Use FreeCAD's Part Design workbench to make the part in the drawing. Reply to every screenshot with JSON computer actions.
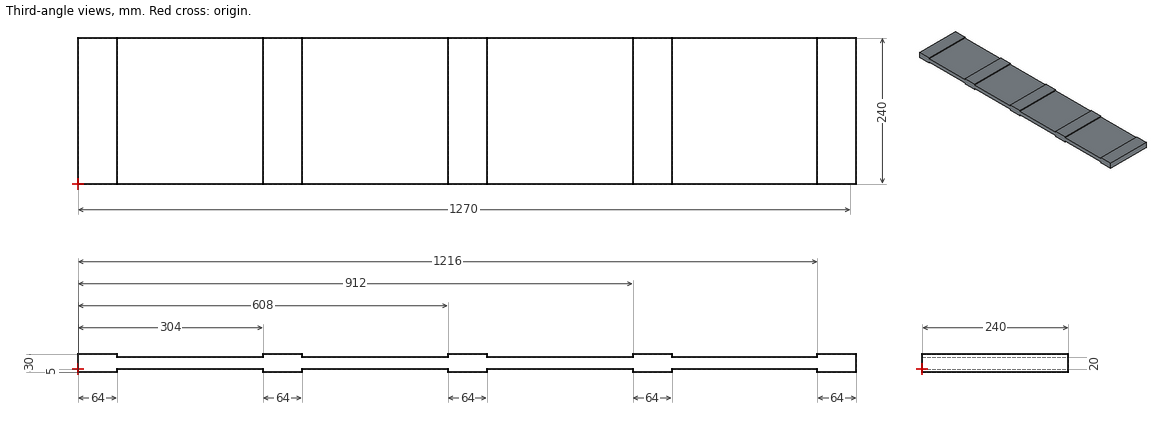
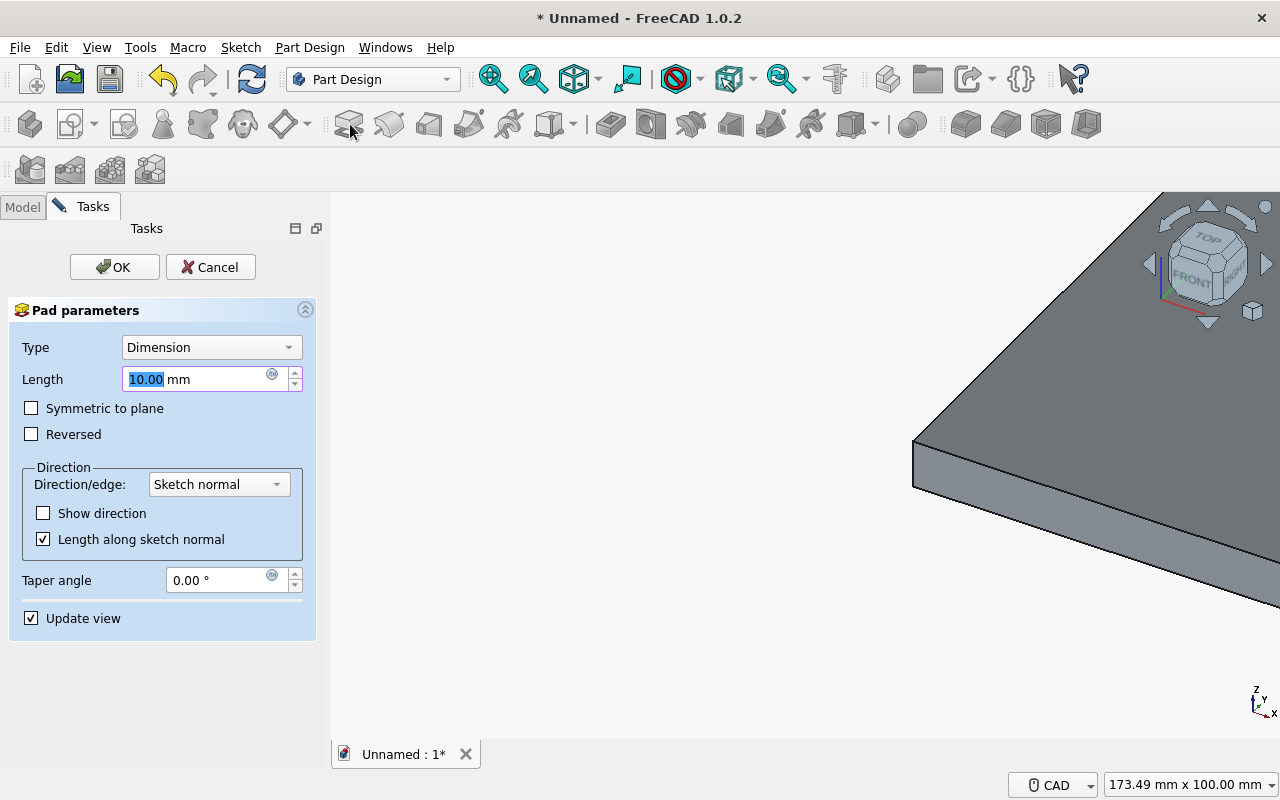
{"action": "type", "text": "20"}
{"action": "key", "text": "Tab"}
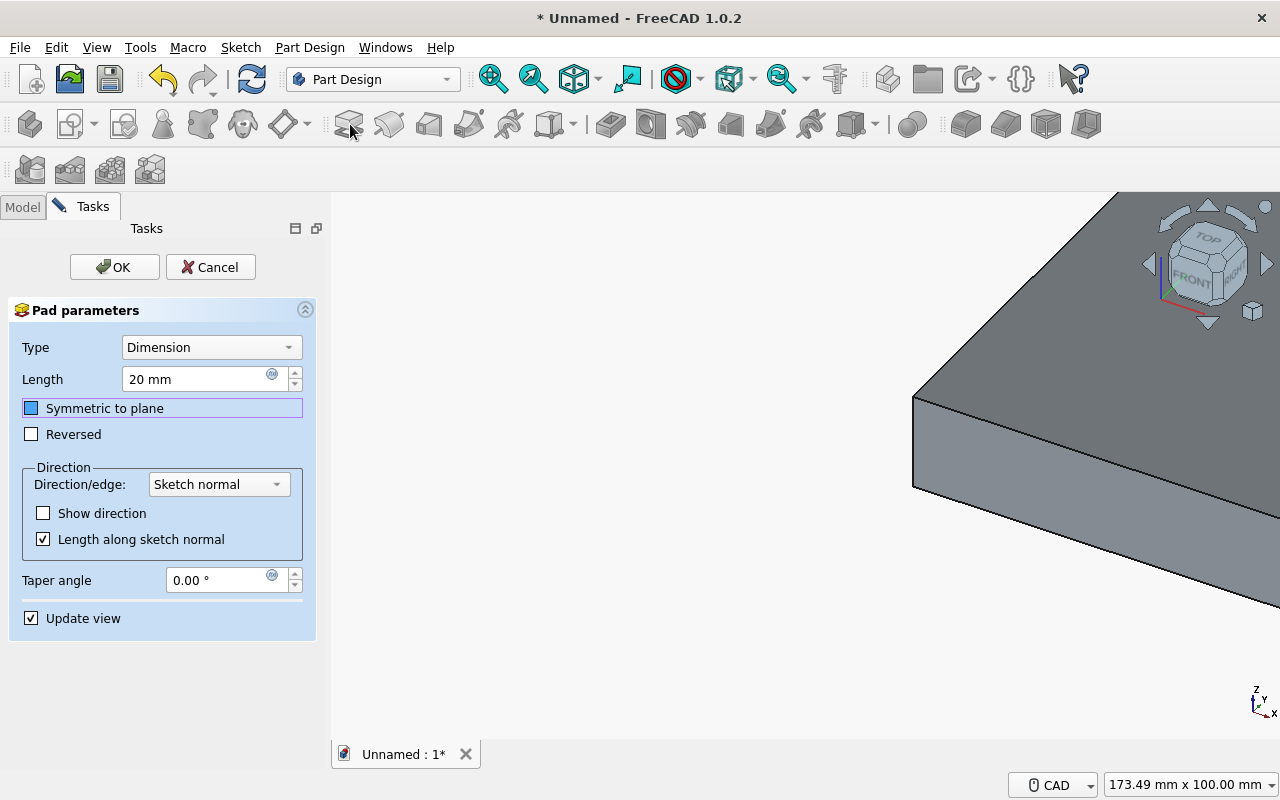
{"action": "left_click", "coordinate": [115, 267]}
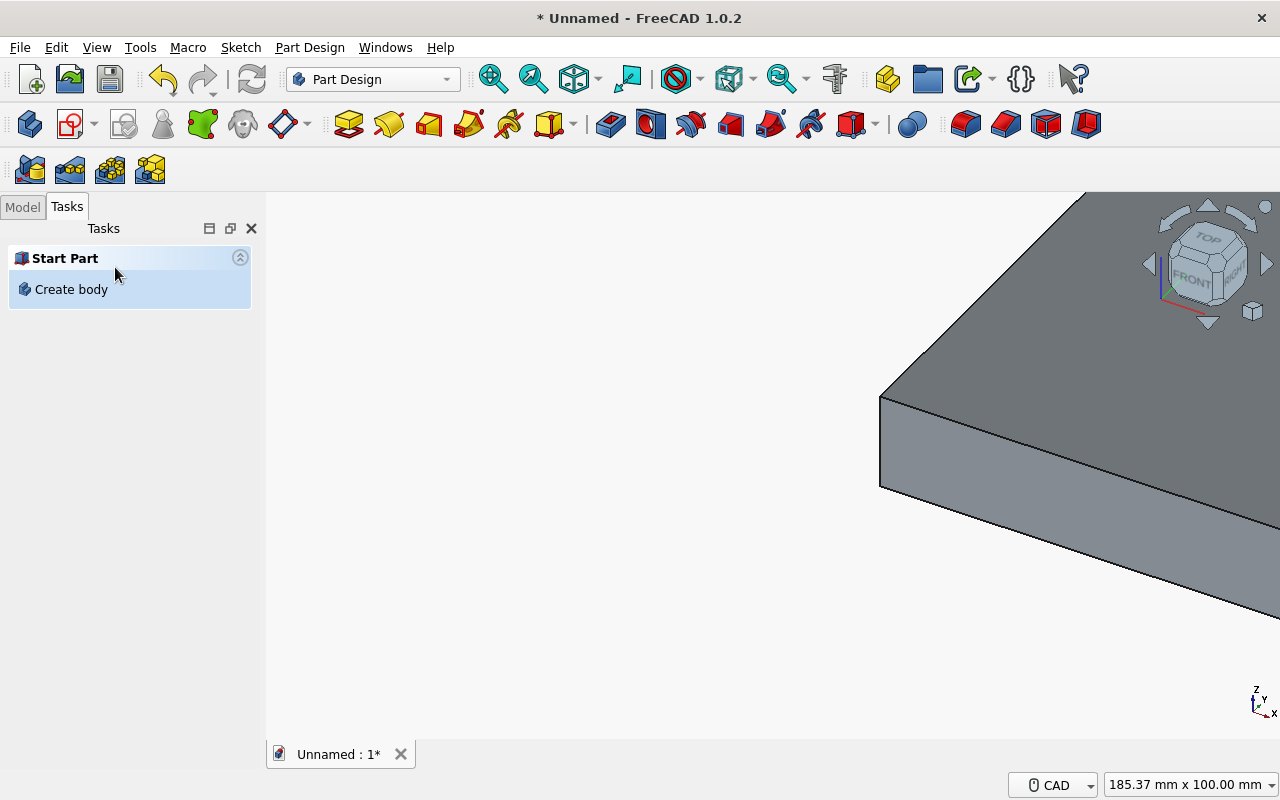
{"action": "left_click", "coordinate": [494, 80]}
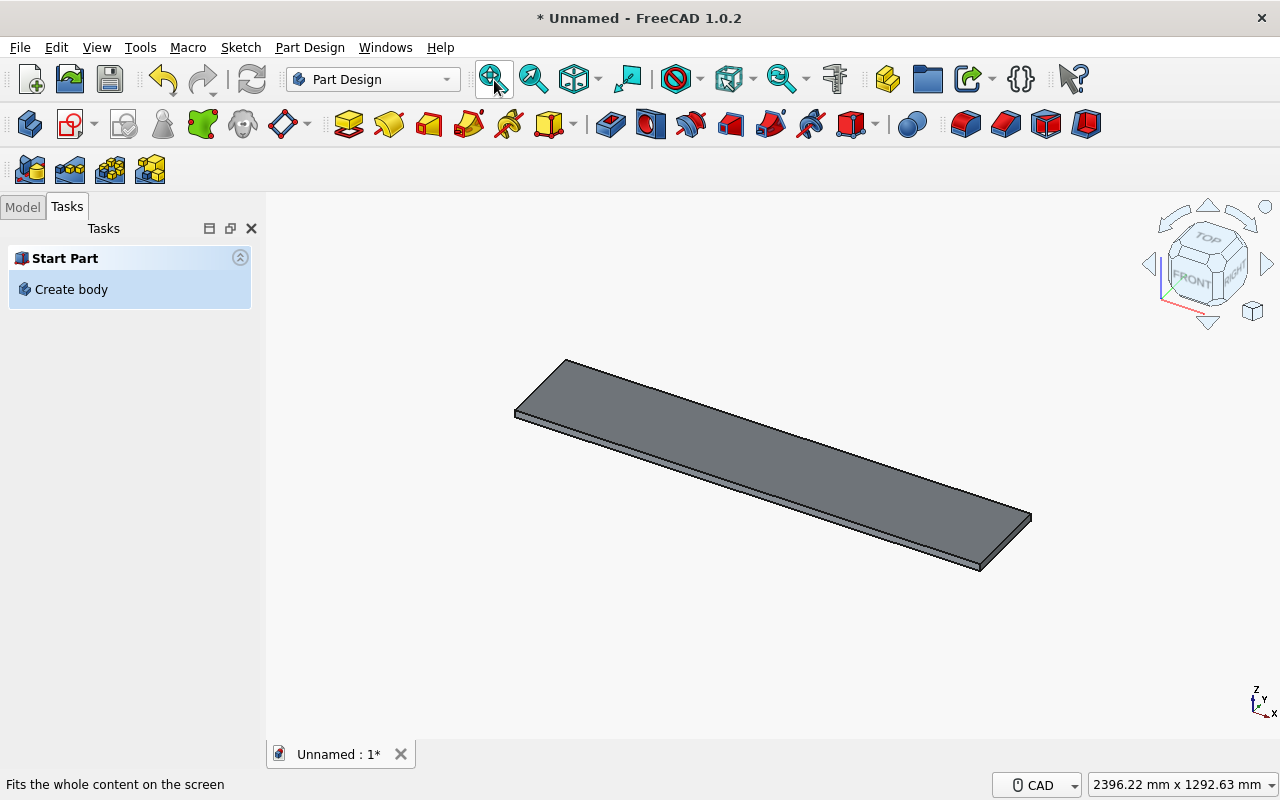
{"action": "scroll", "coordinate": [947, 556], "scroll_direction": "up", "scroll_amount": 6}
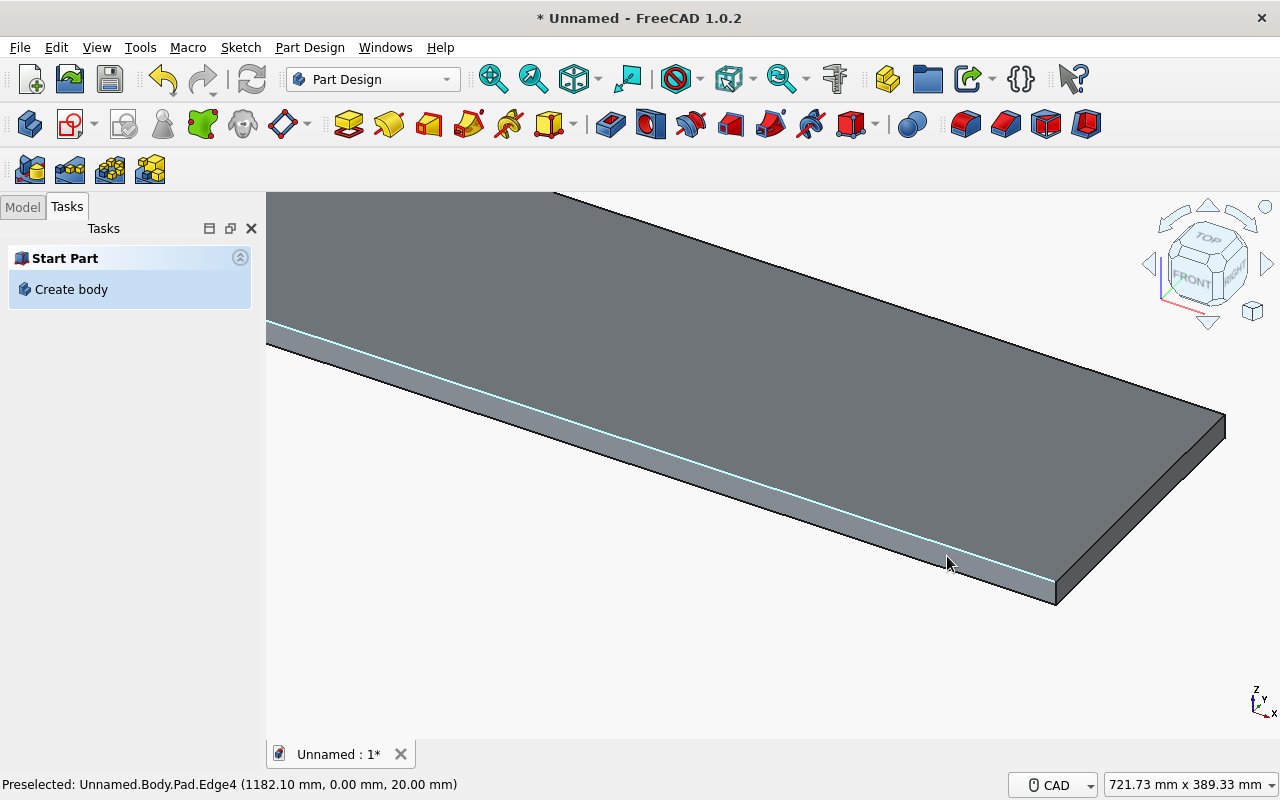
{"action": "left_click", "coordinate": [946, 556]}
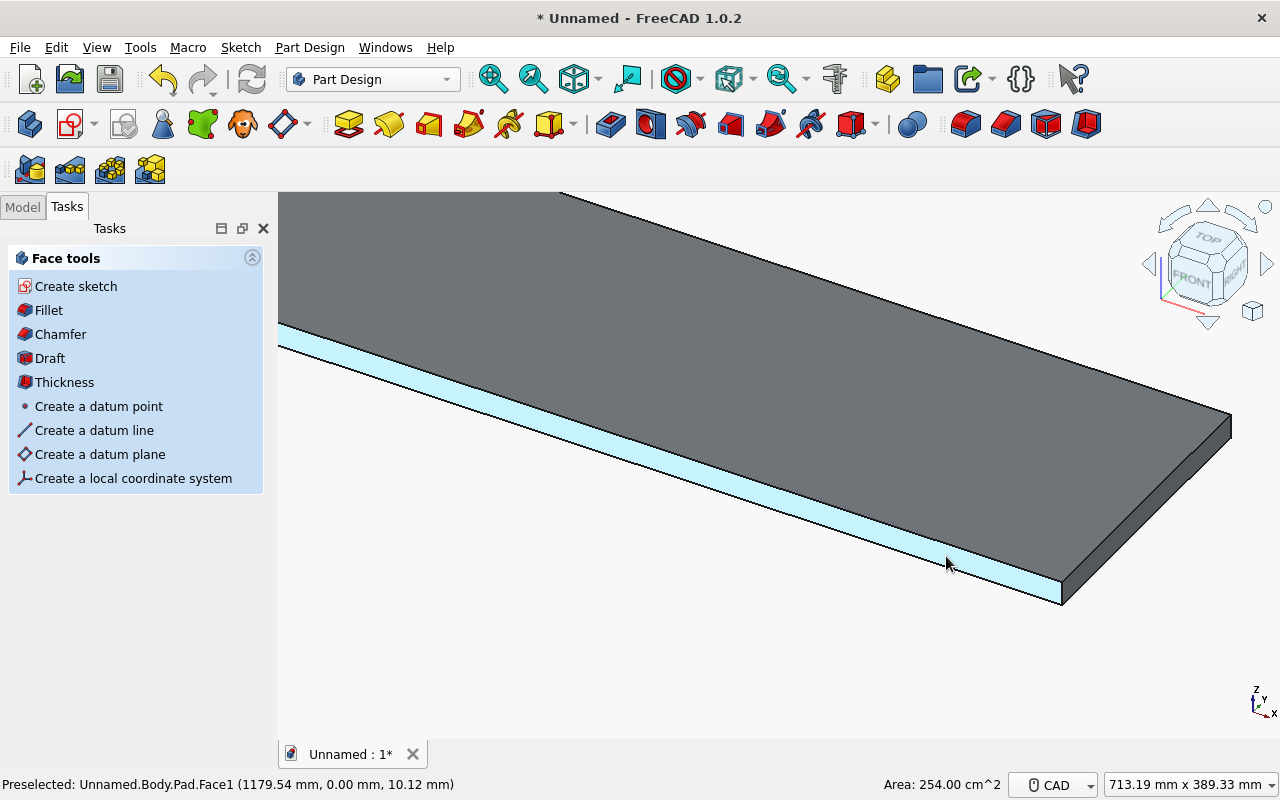
{"action": "left_click", "coordinate": [70, 124]}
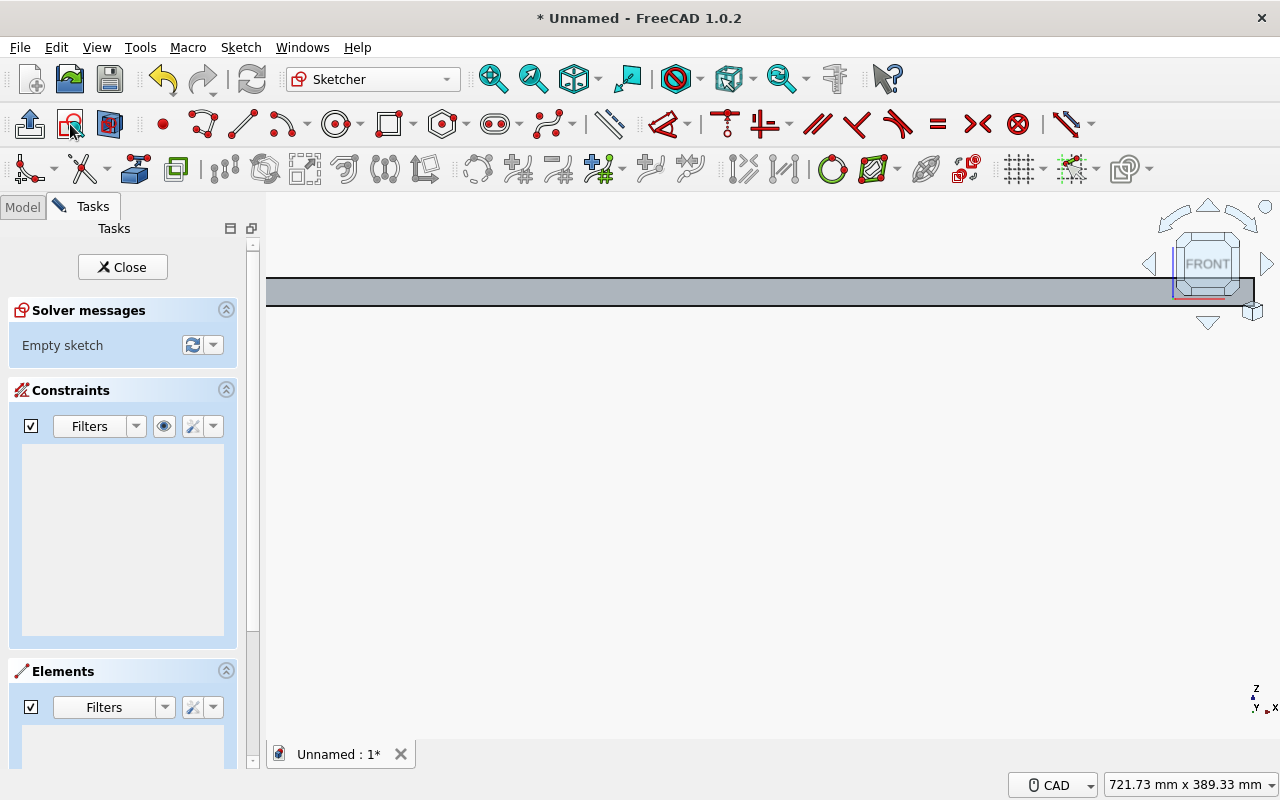
{"action": "scroll", "coordinate": [849, 540], "scroll_direction": "down", "scroll_amount": 6}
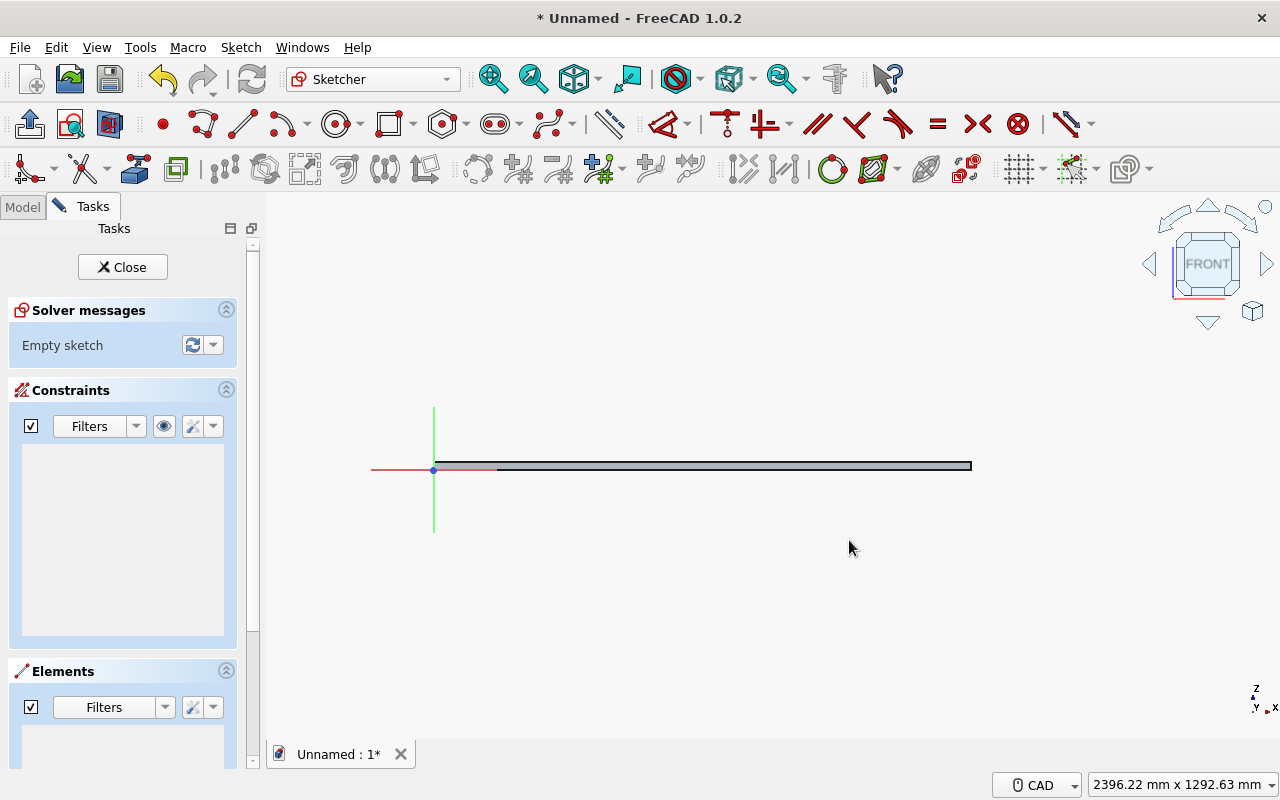
{"action": "left_click", "coordinate": [390, 124]}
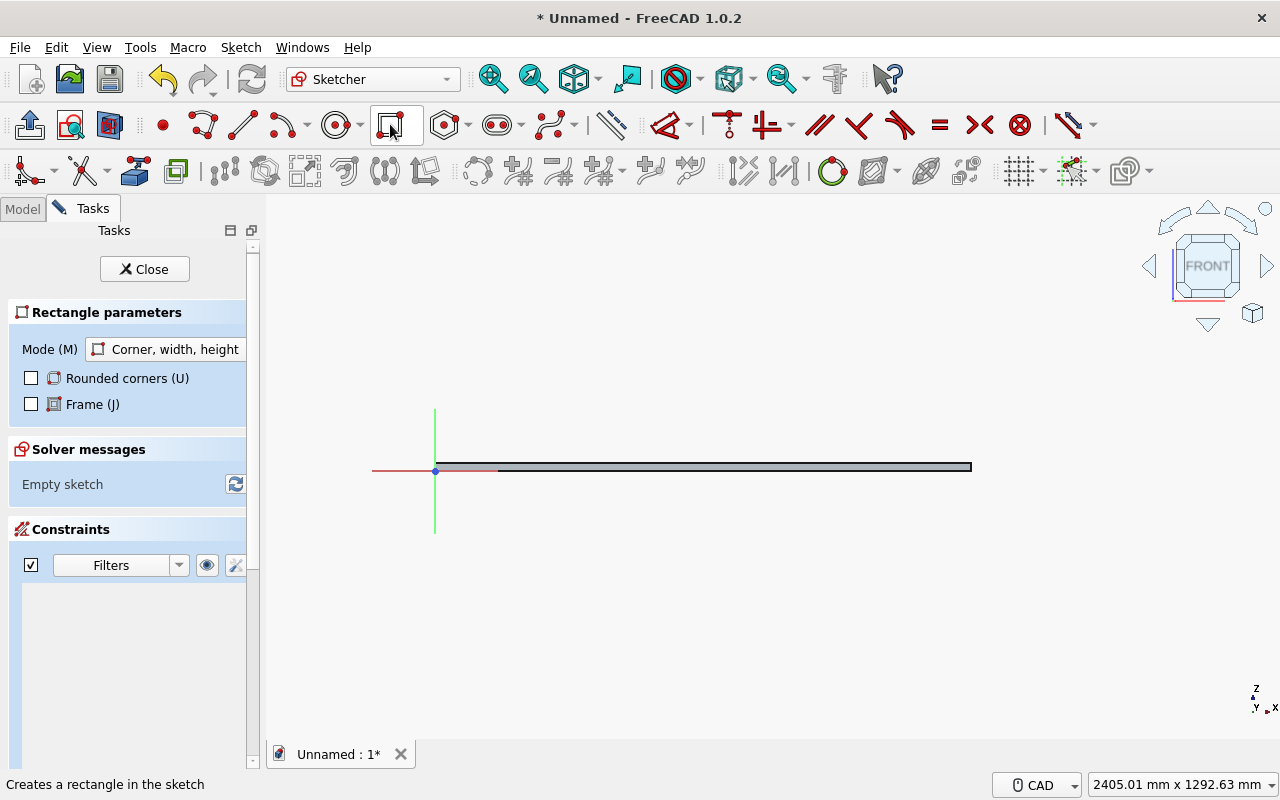
{"action": "scroll", "coordinate": [435, 460], "scroll_direction": "up", "scroll_amount": 3}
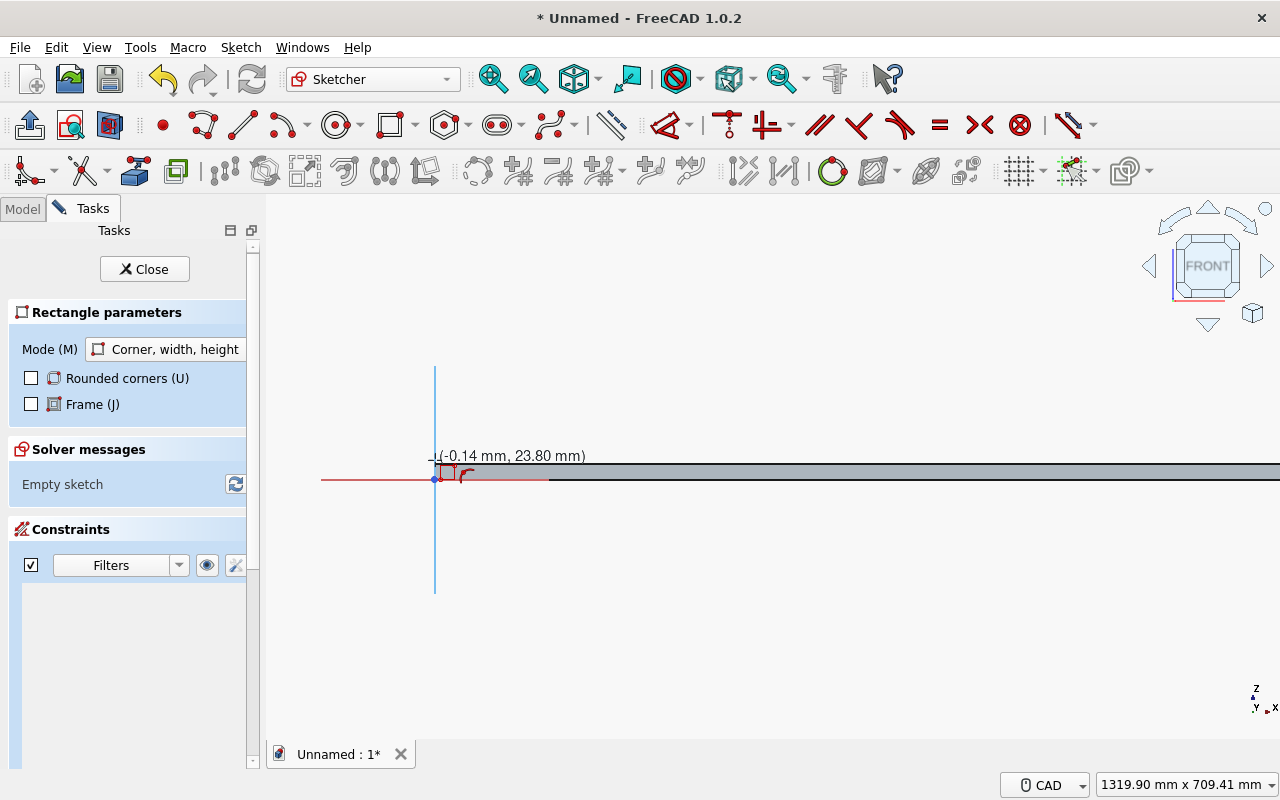
{"action": "left_click", "coordinate": [435, 460]}